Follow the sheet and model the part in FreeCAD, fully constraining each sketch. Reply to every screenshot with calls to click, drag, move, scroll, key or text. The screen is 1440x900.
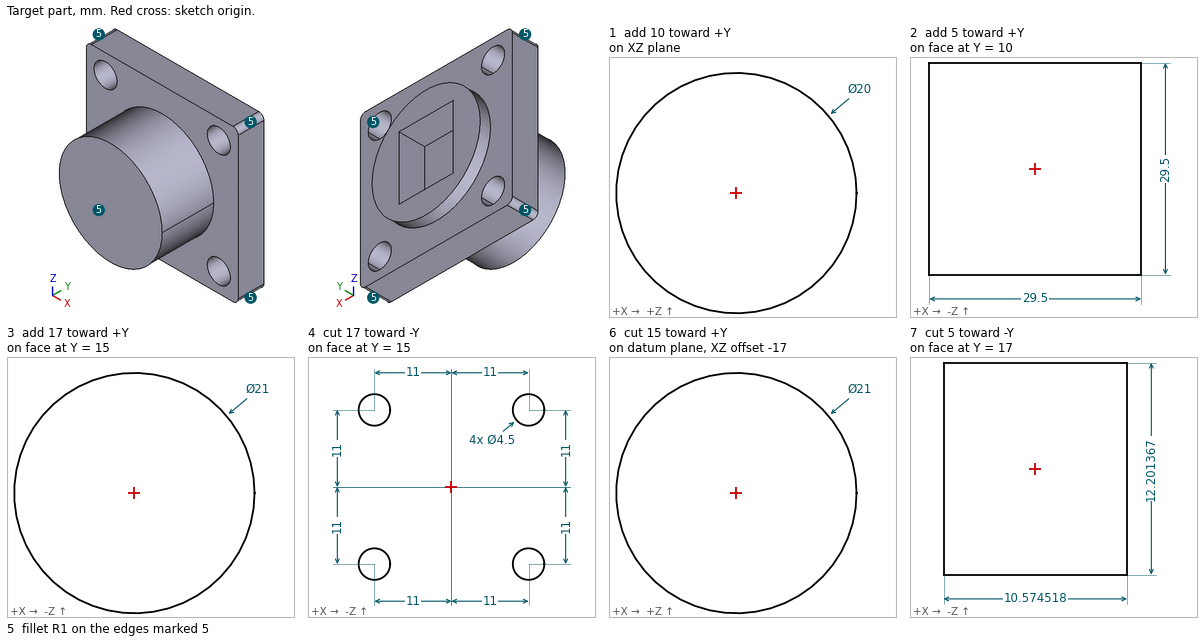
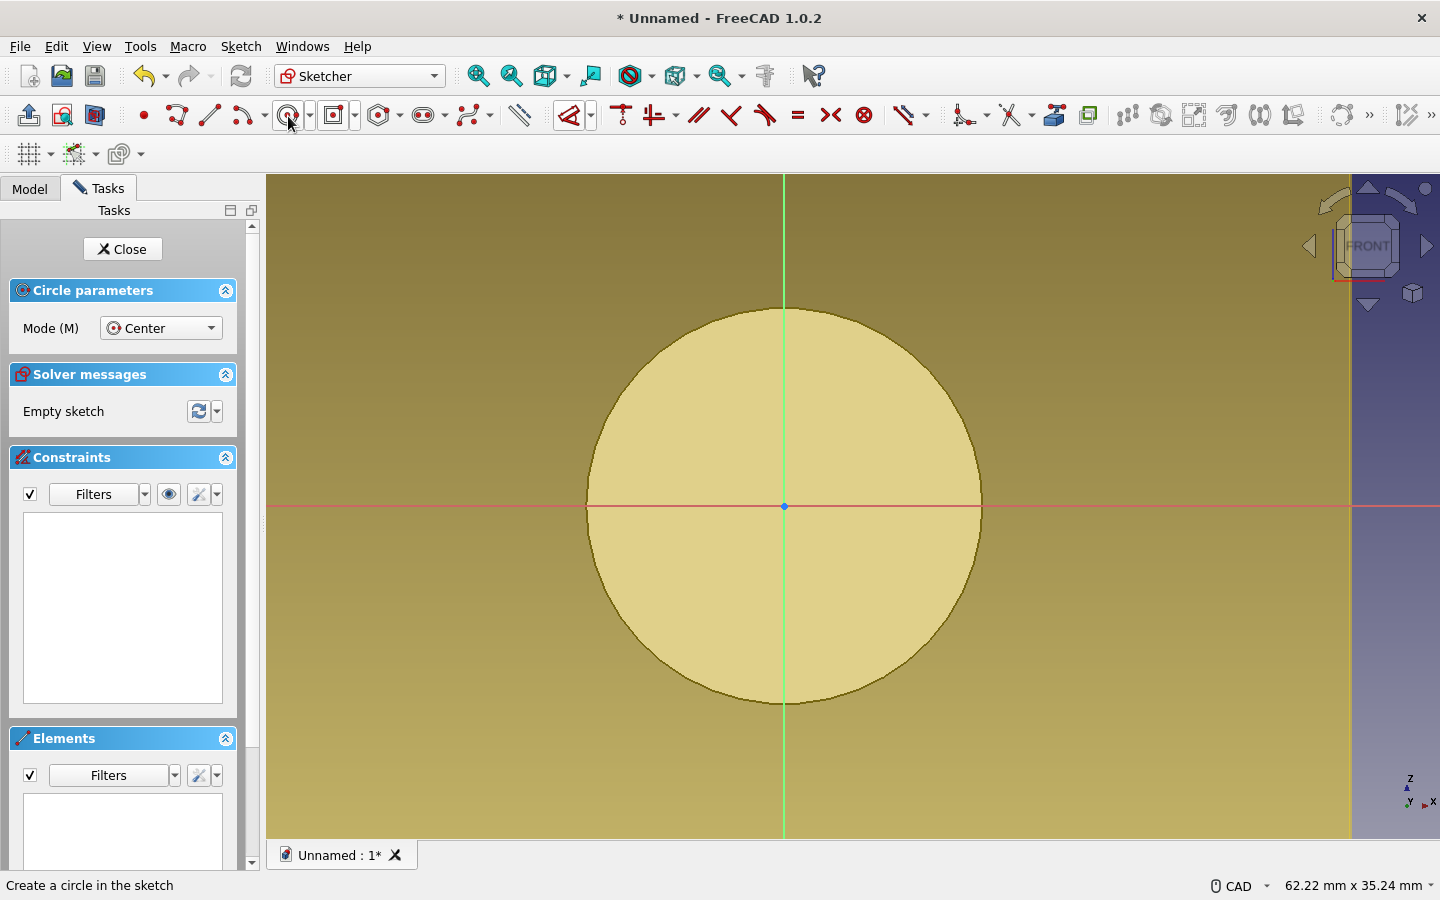
click(784, 506)
click(924, 366)
key(Escape)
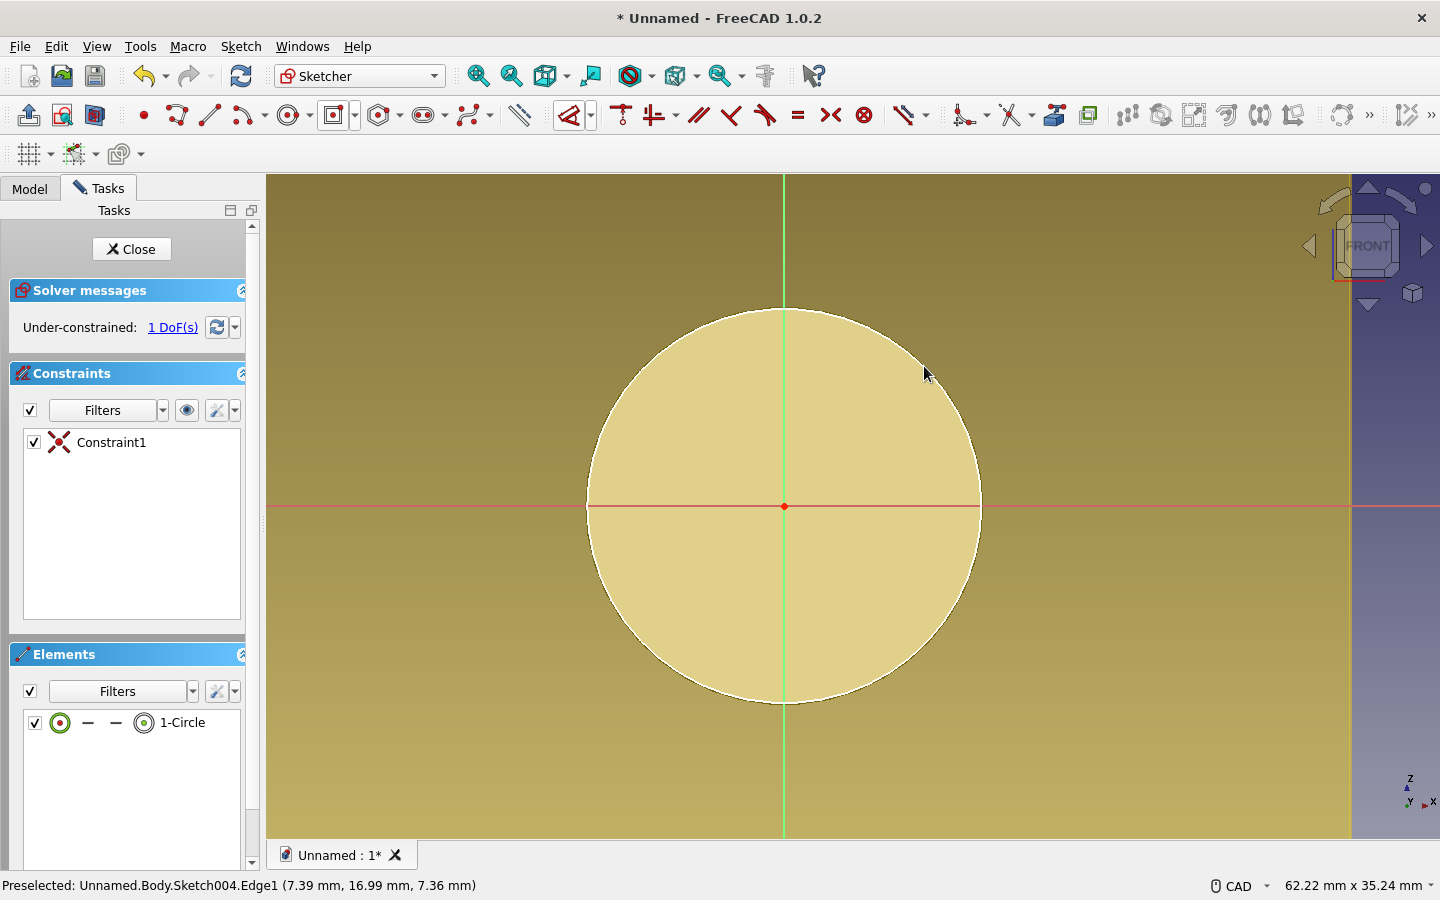
click(923, 366)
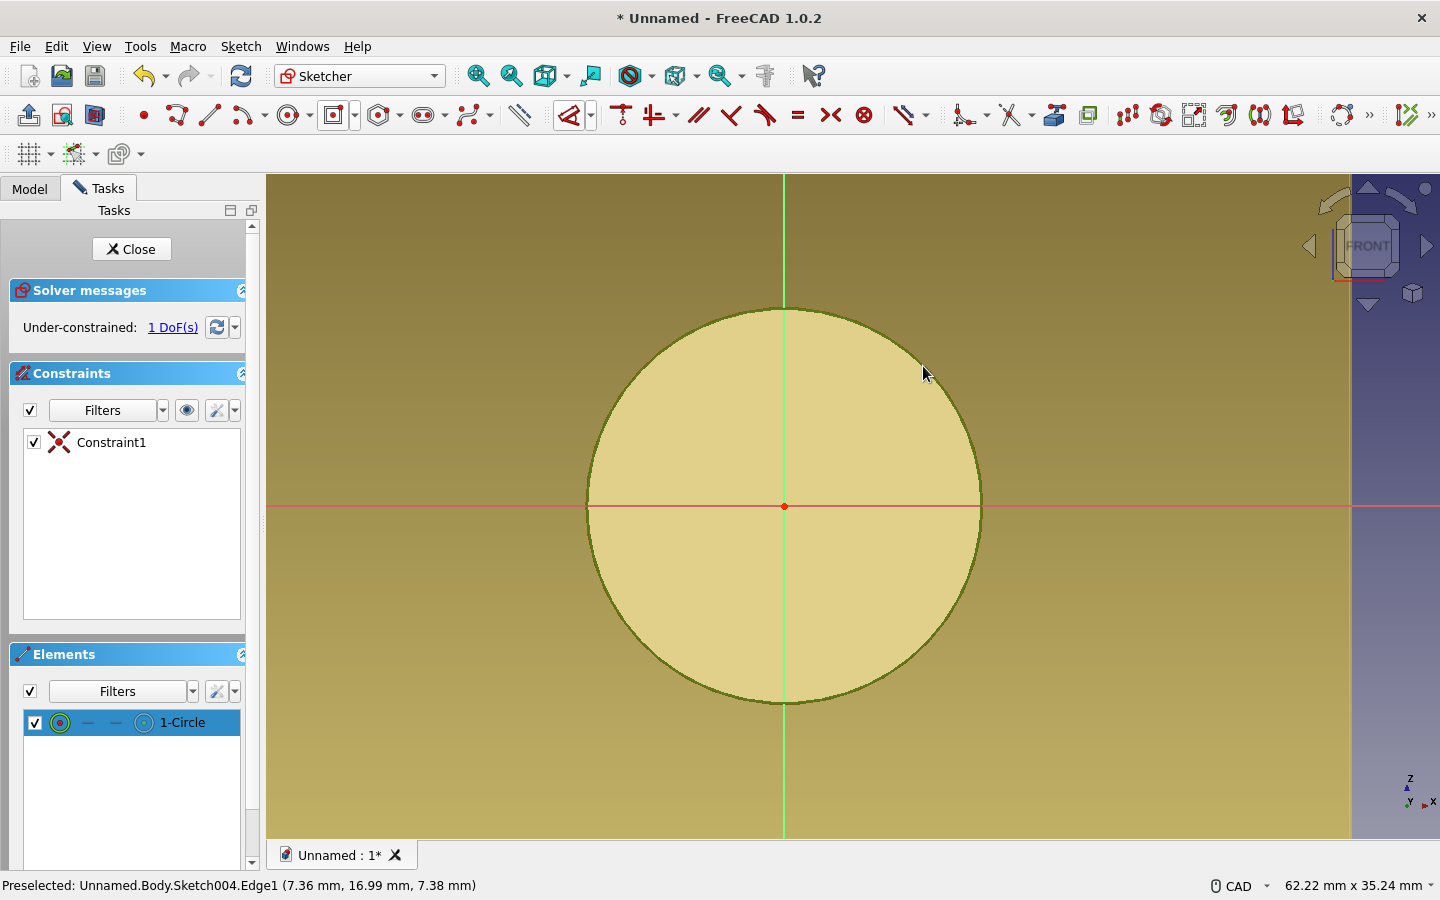
click(590, 116)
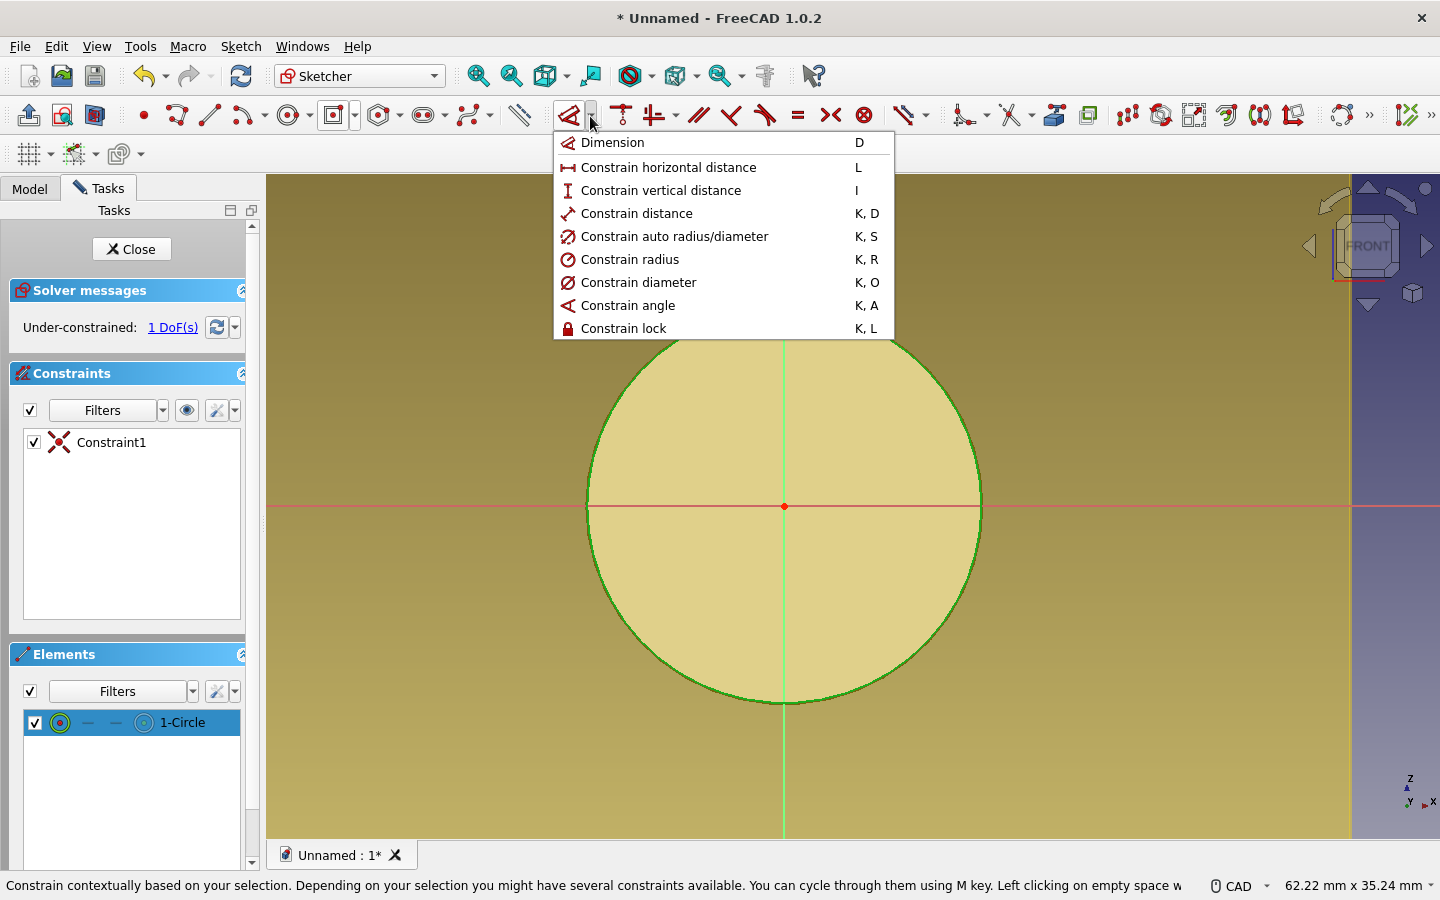
click(724, 282)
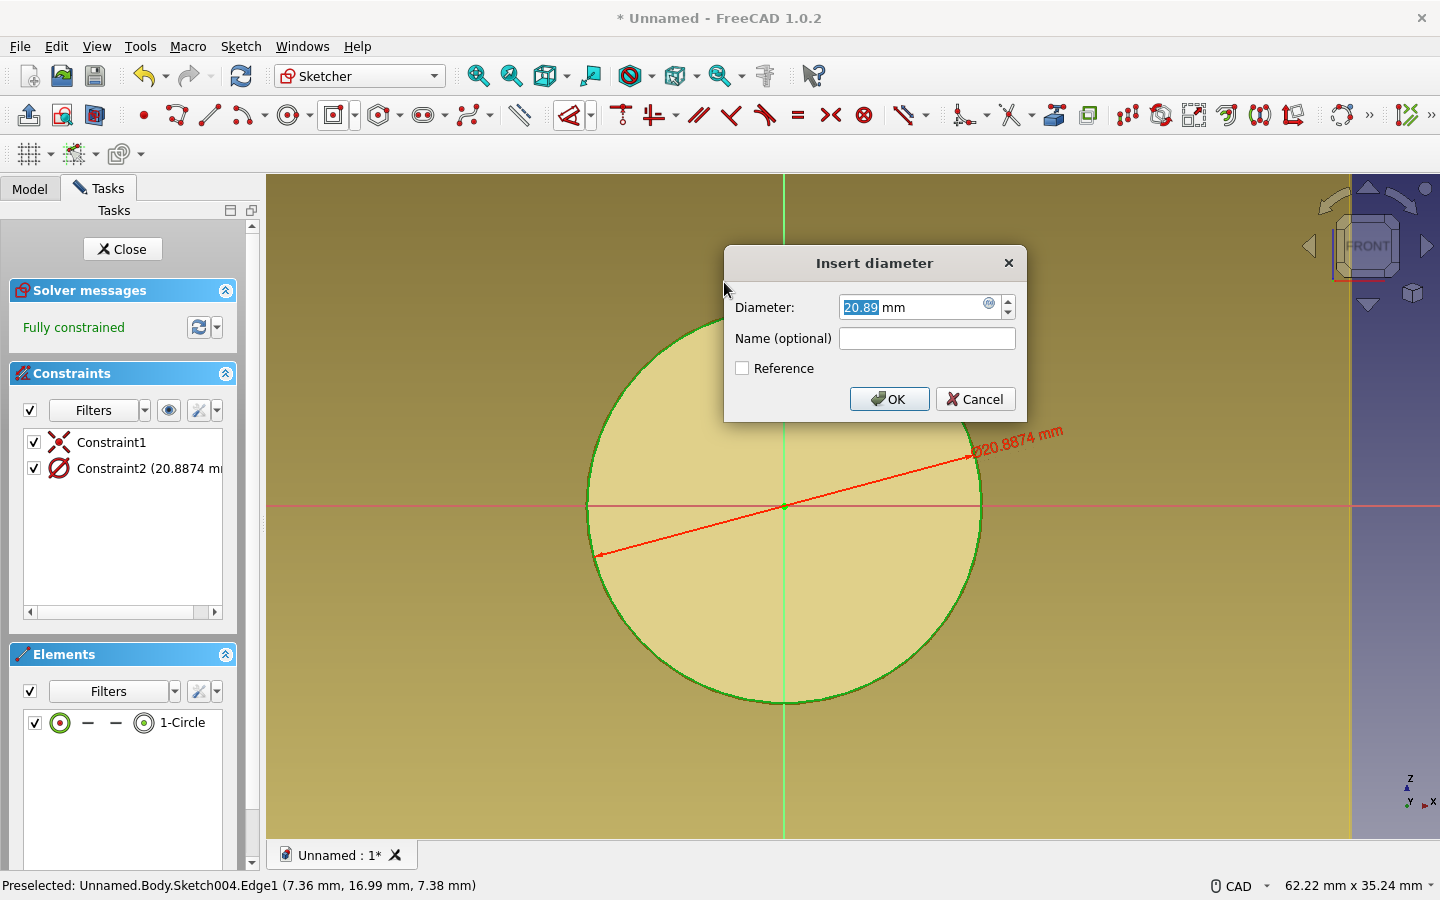
text(21)
key(Return)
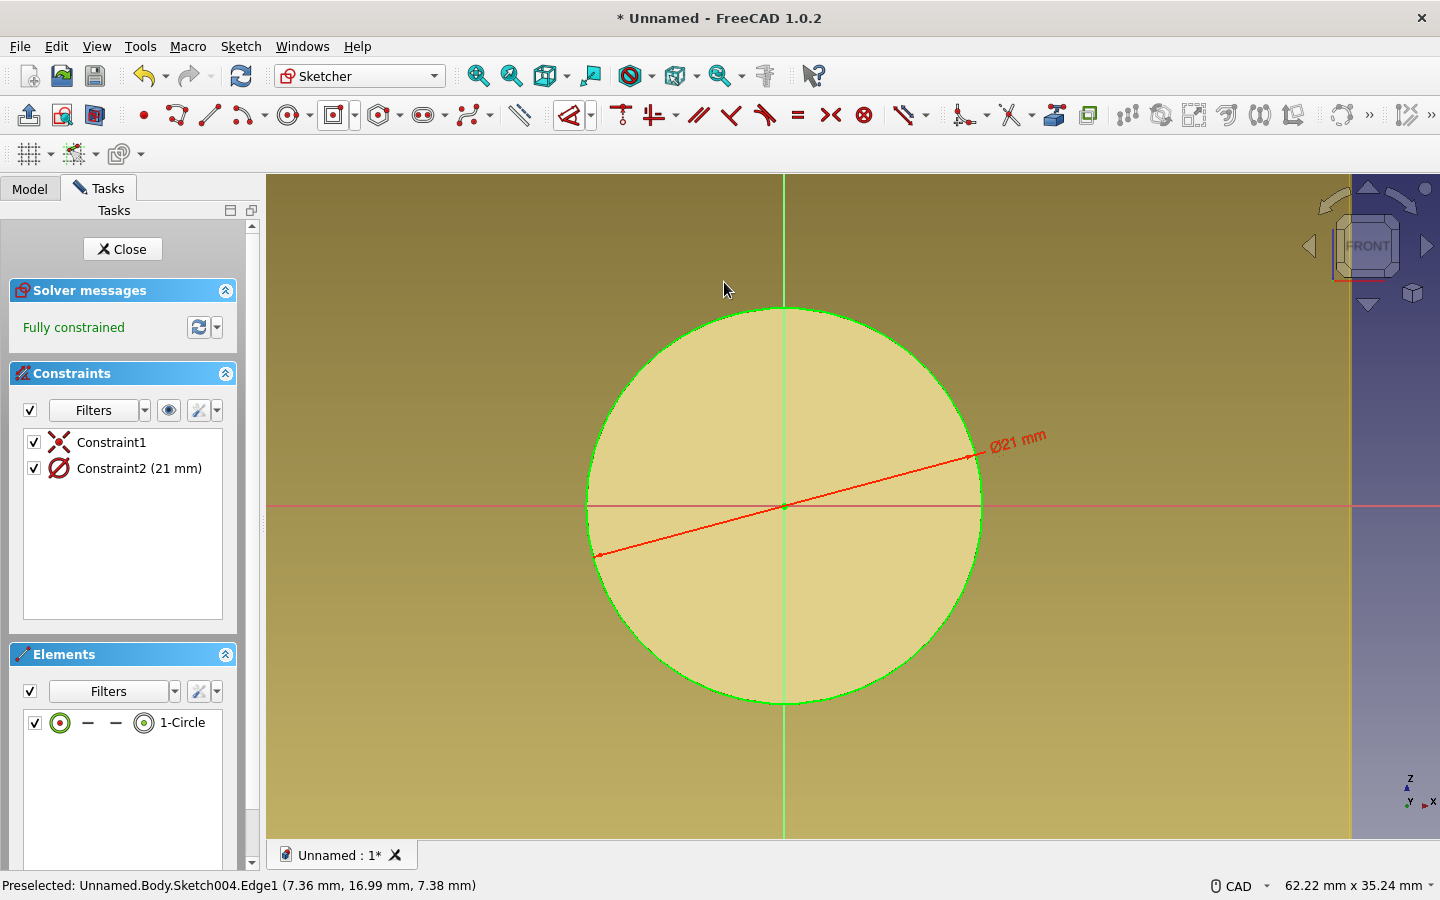
click(123, 249)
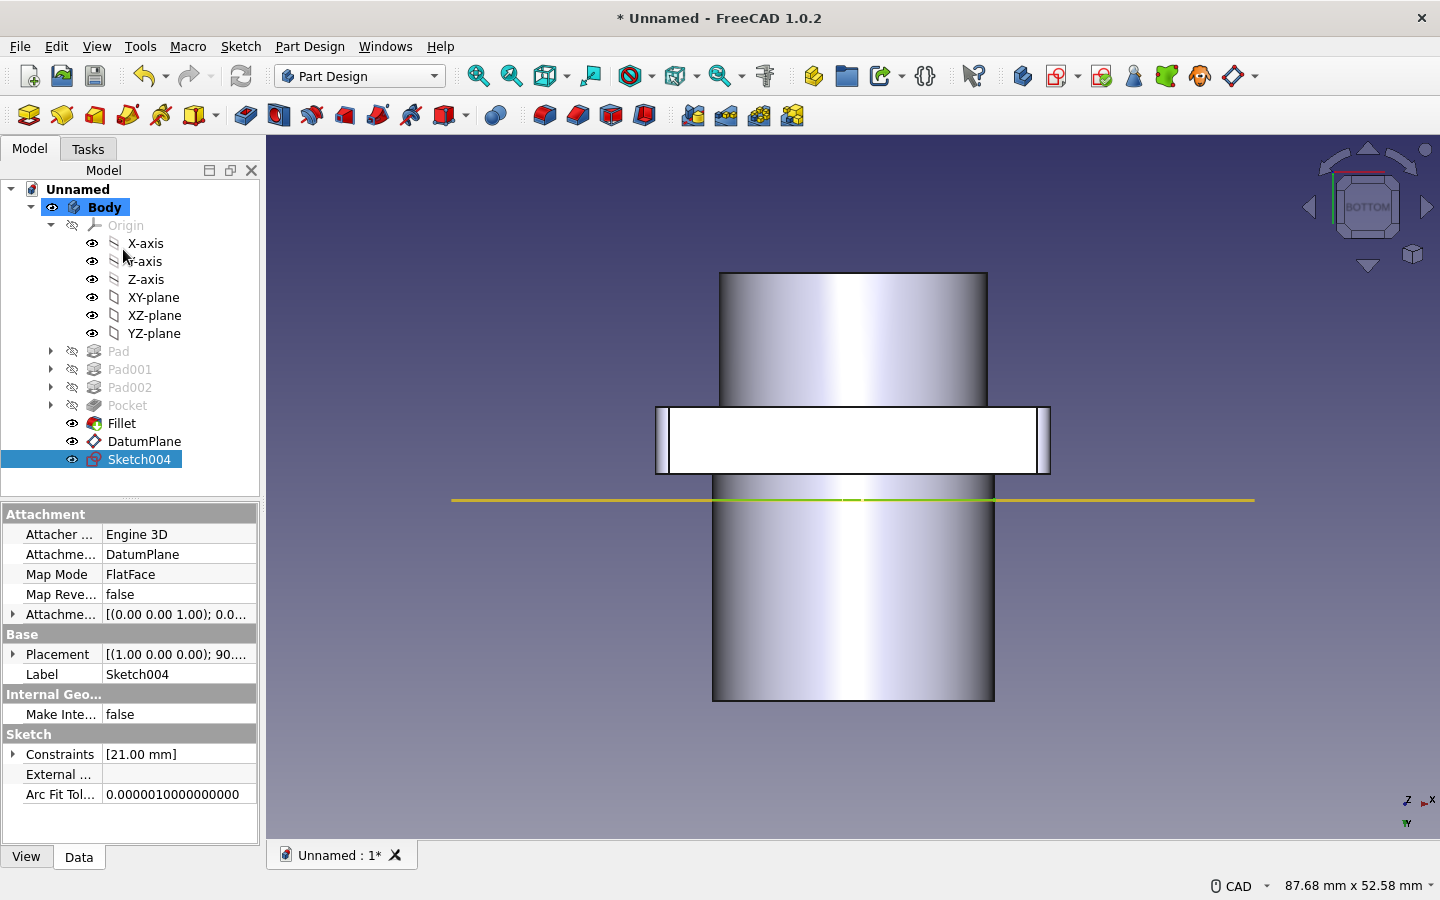
click(246, 116)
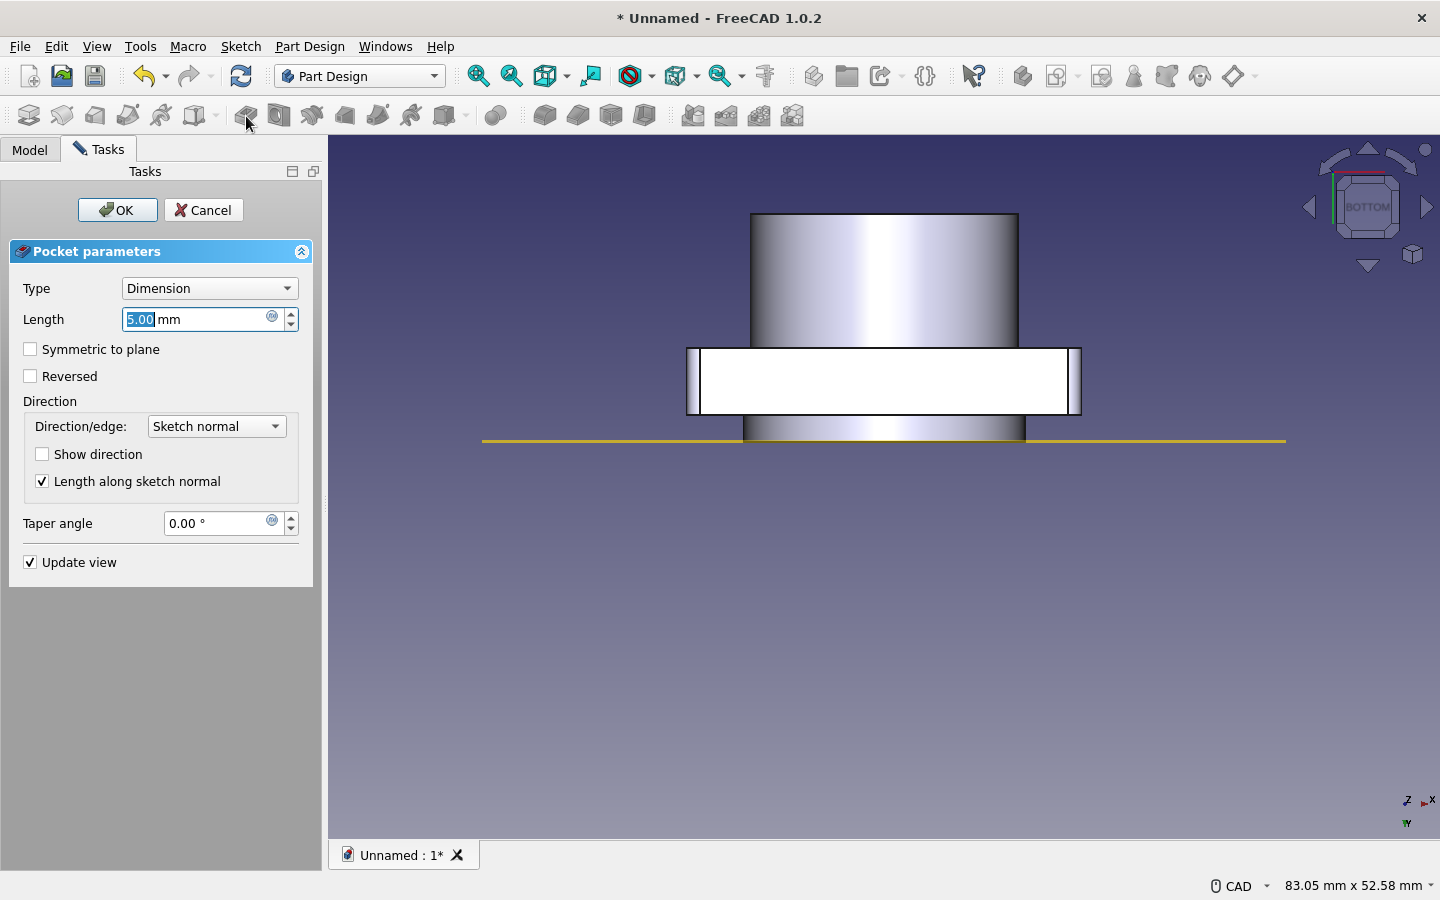
text(15)
key(Tab)